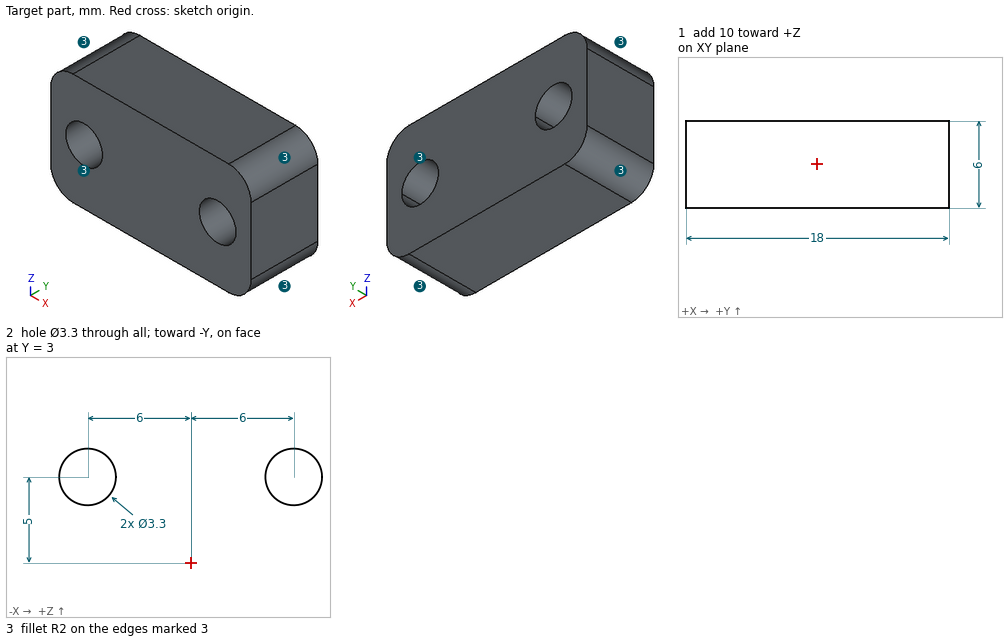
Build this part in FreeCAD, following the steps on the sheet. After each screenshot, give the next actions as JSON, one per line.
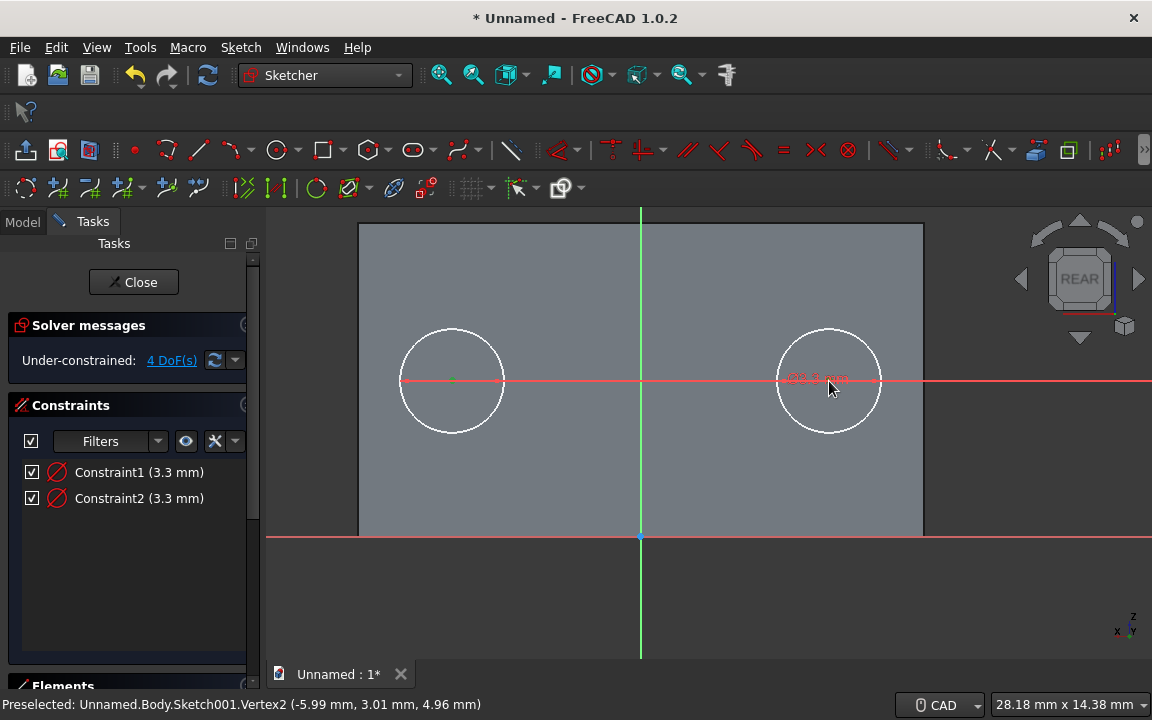
{"action": "left_click", "coordinate": [666, 150]}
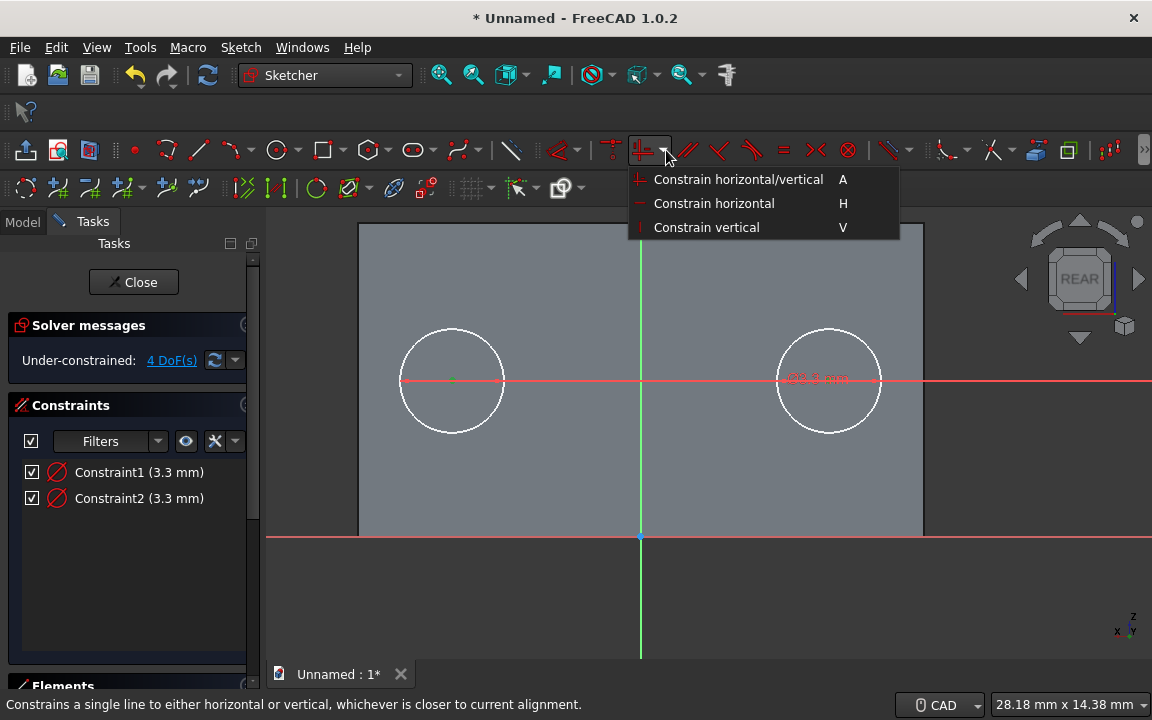
{"action": "left_click", "coordinate": [764, 203]}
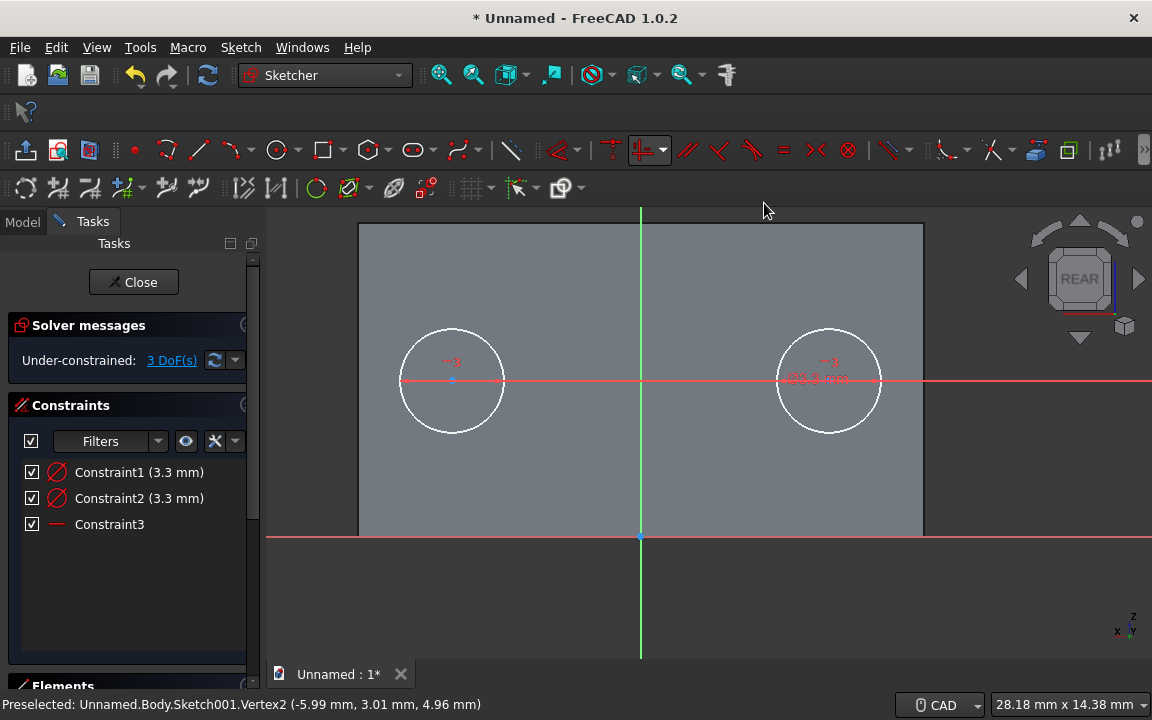
{"action": "left_click", "coordinate": [558, 150]}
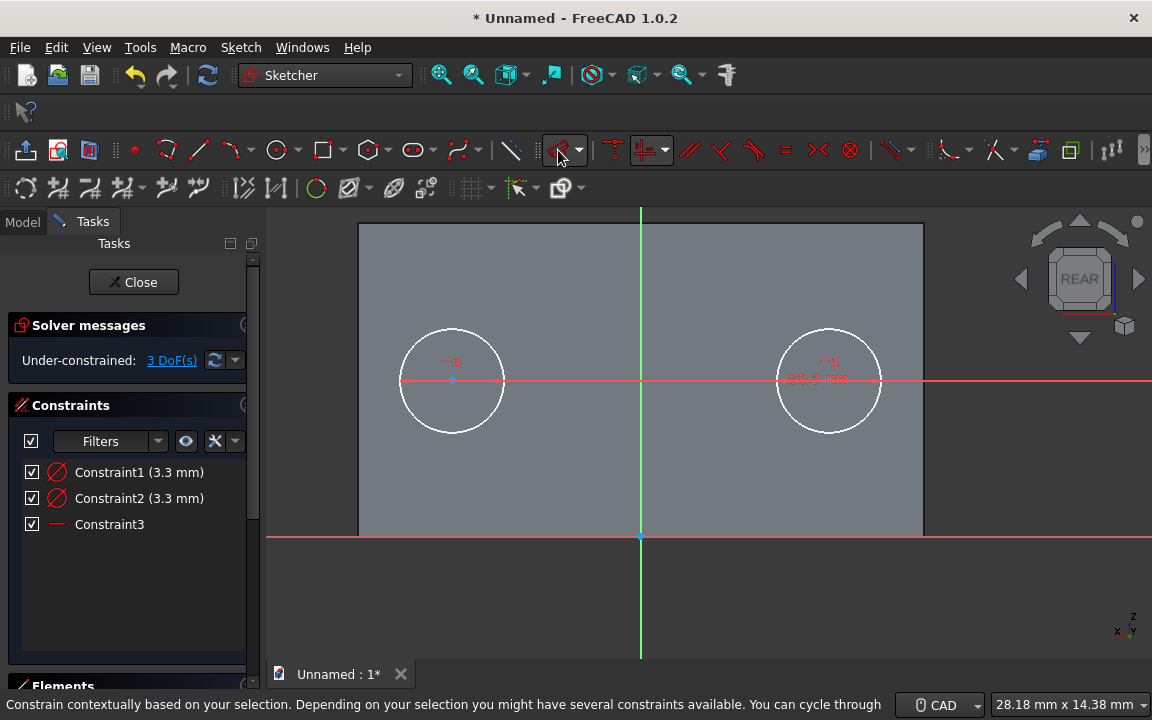
{"action": "left_click", "coordinate": [452, 381]}
{"action": "left_click", "coordinate": [546, 571]}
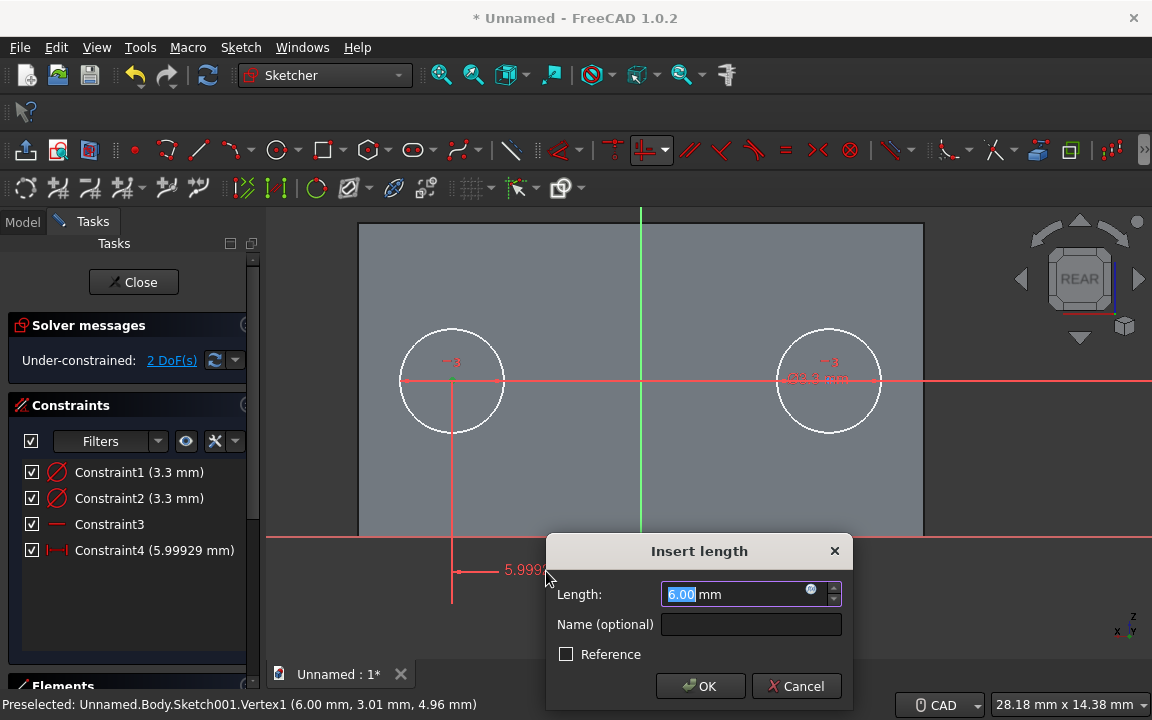
{"action": "type", "text": "6"}
{"action": "key", "text": "Return"}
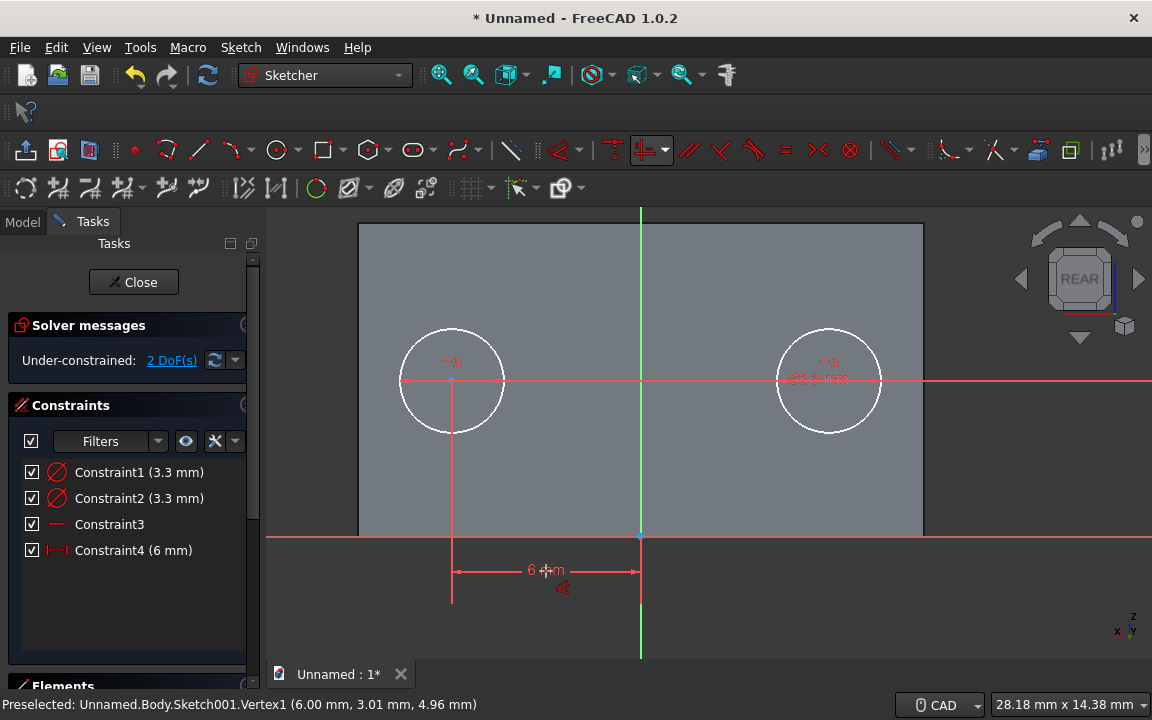
{"action": "left_click", "coordinate": [452, 381]}
{"action": "left_click", "coordinate": [418, 459]}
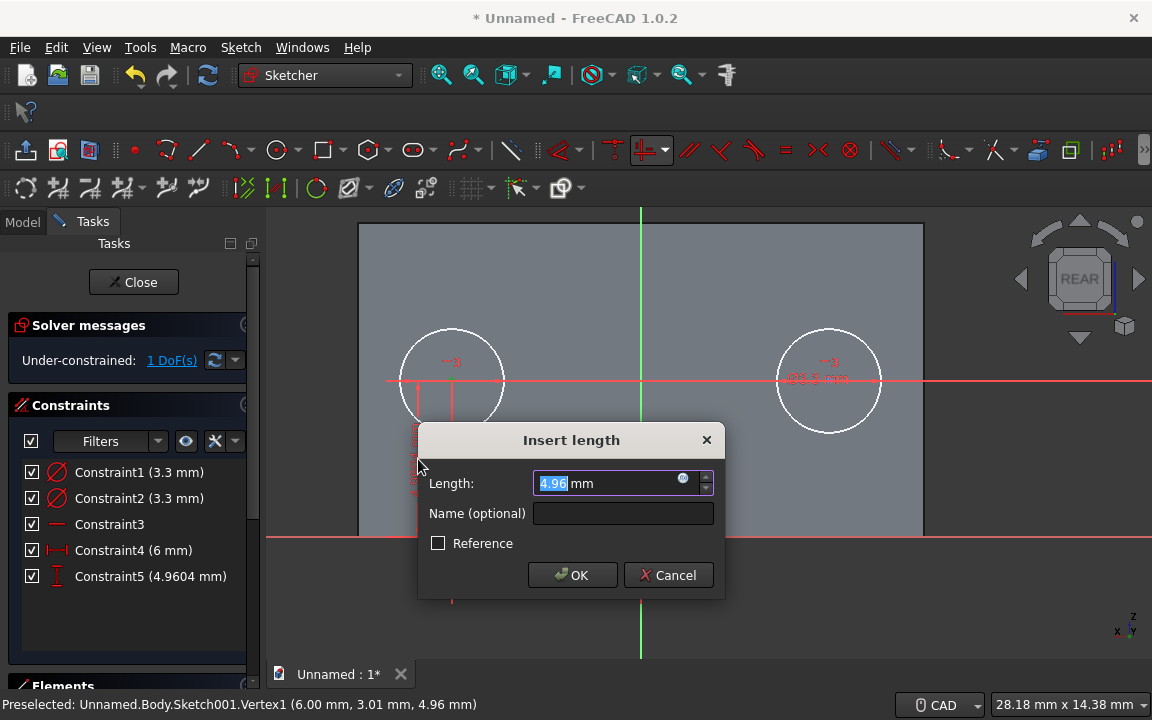
{"action": "type", "text": "5"}
{"action": "key", "text": "Return"}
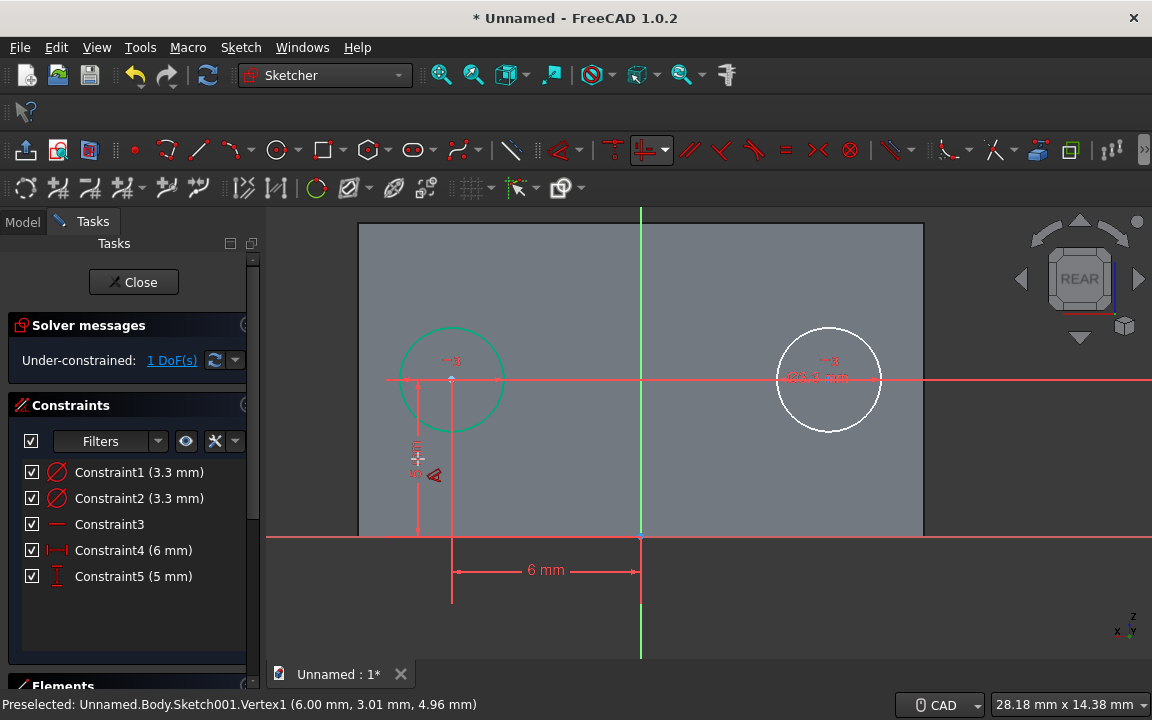
{"action": "left_click", "coordinate": [829, 380]}
{"action": "left_click", "coordinate": [735, 571]}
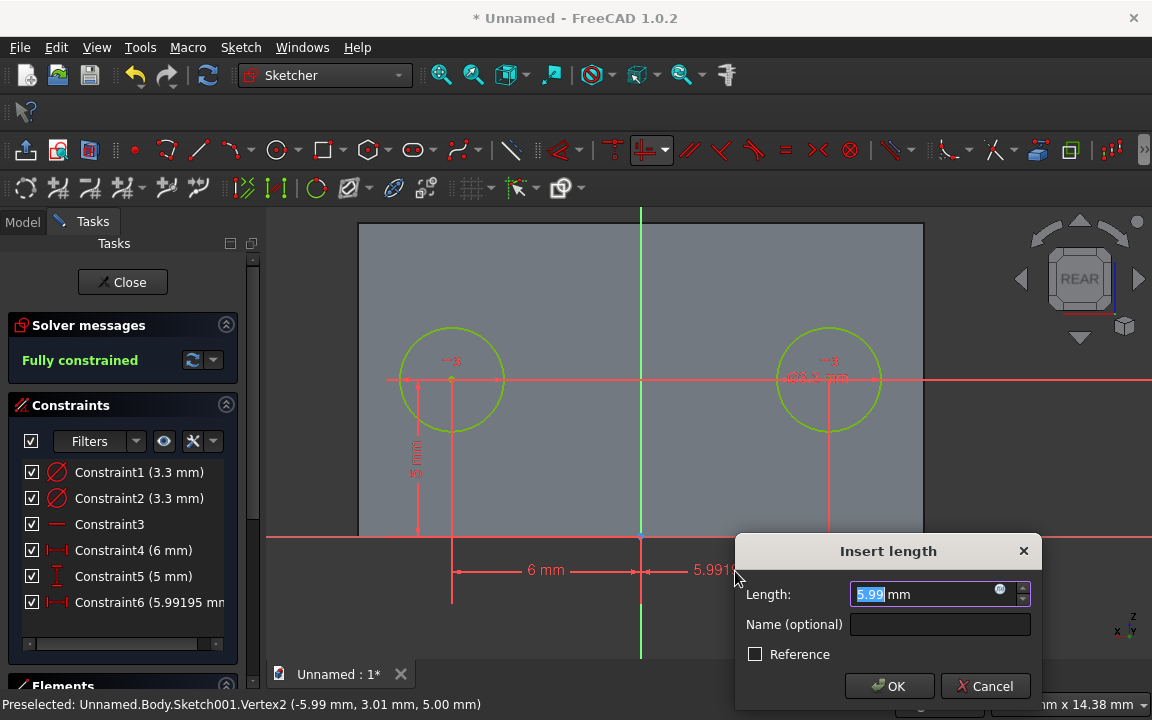
{"action": "type", "text": "6"}
{"action": "key", "text": "Return"}
{"action": "key", "text": "Escape"}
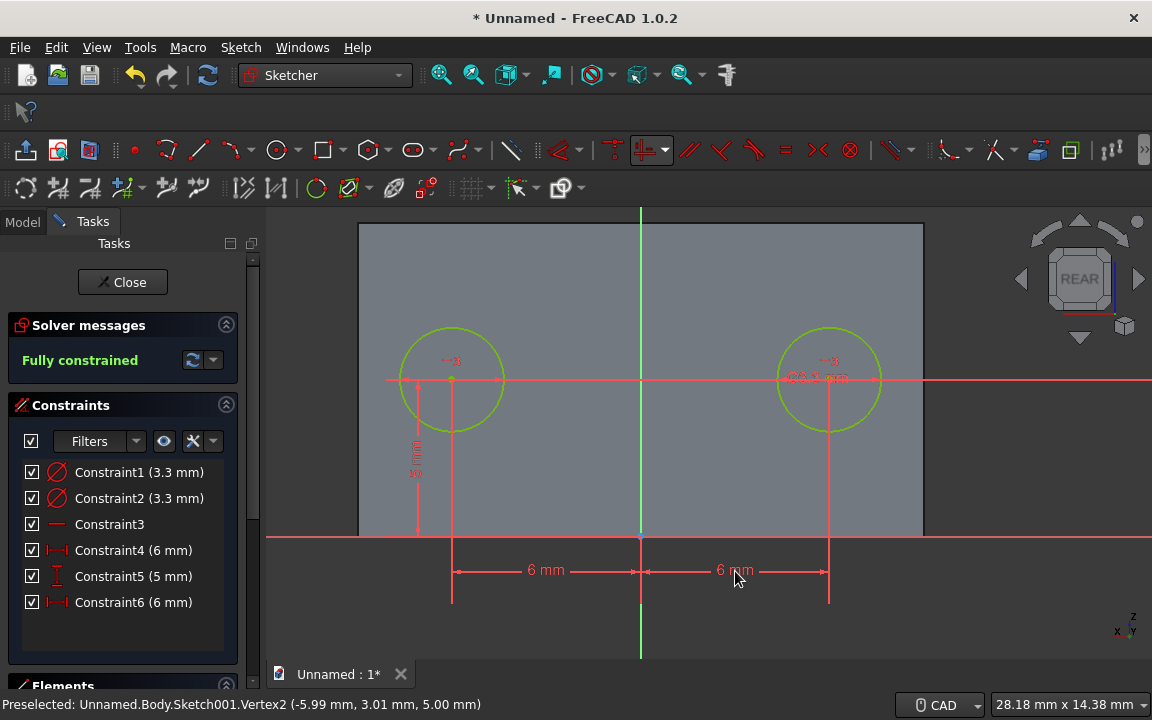
{"action": "left_click", "coordinate": [123, 282]}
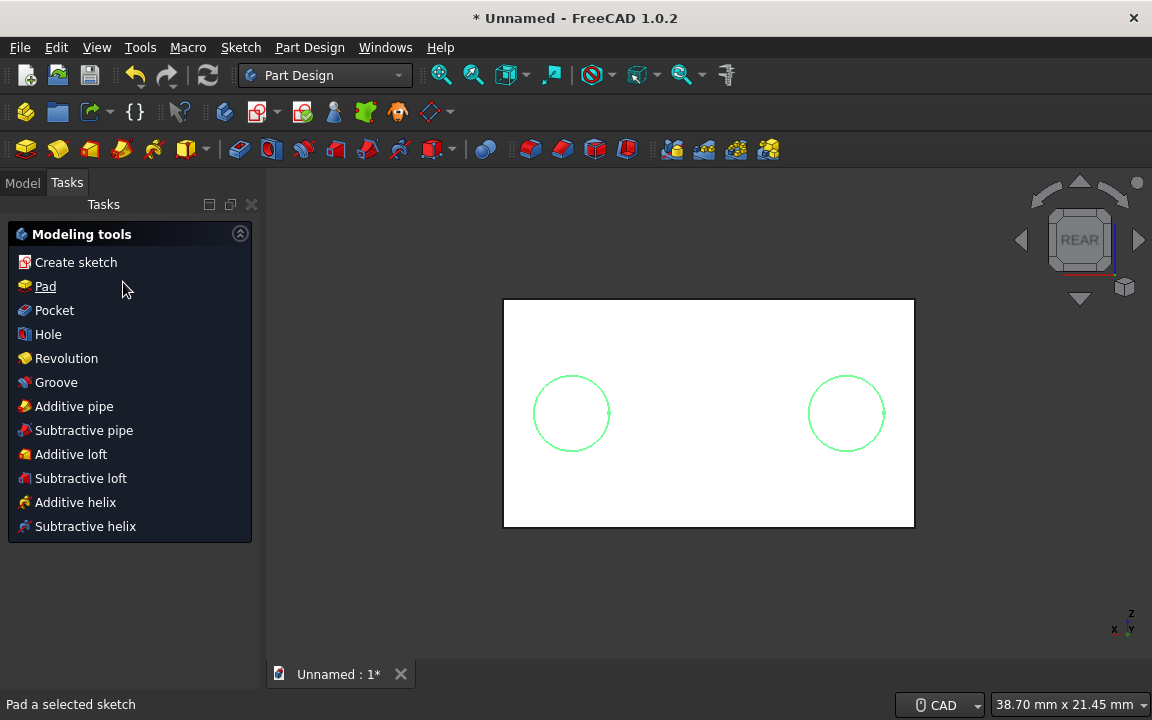
{"action": "left_click", "coordinate": [272, 150]}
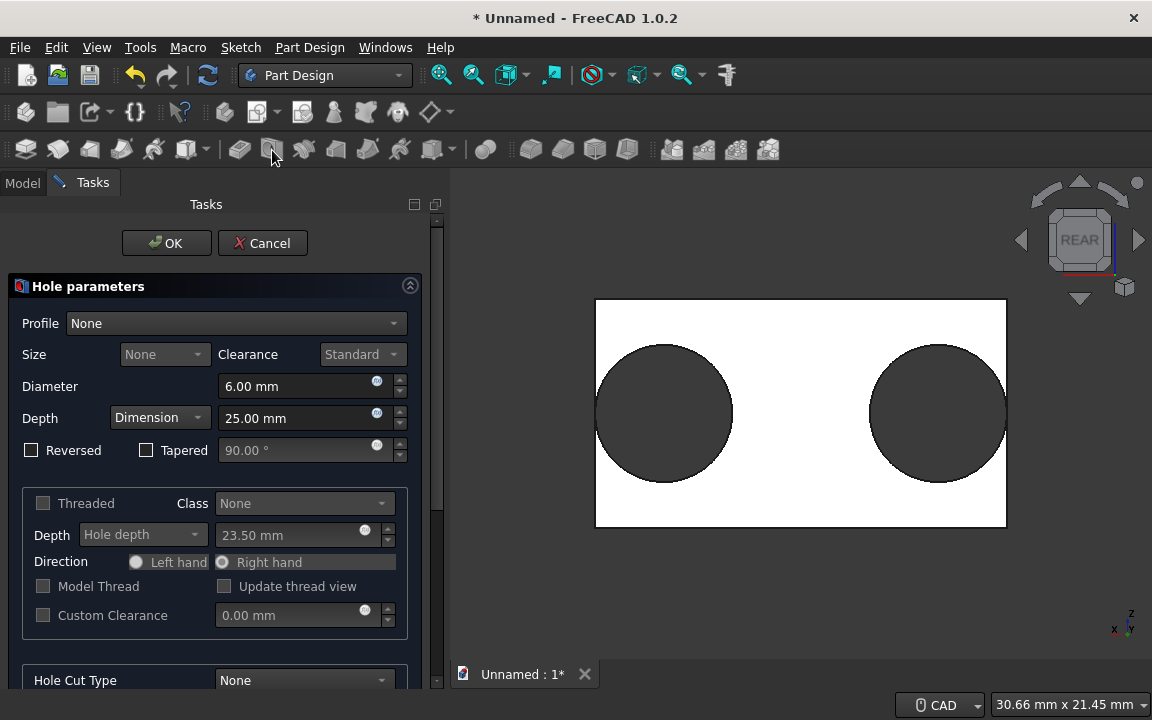
{"action": "triple_click", "coordinate": [305, 386]}